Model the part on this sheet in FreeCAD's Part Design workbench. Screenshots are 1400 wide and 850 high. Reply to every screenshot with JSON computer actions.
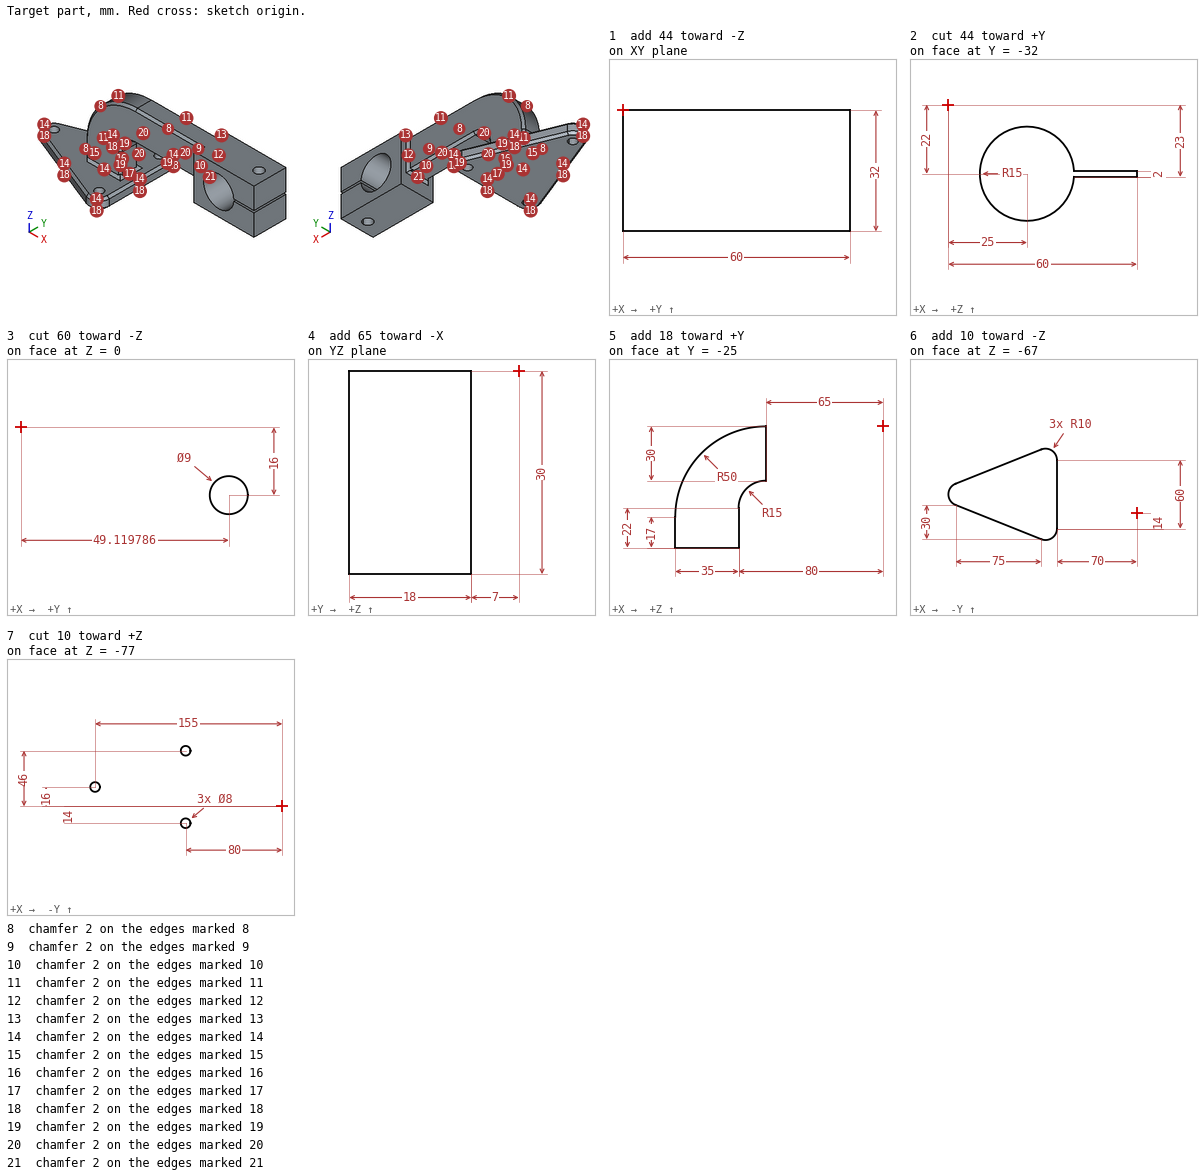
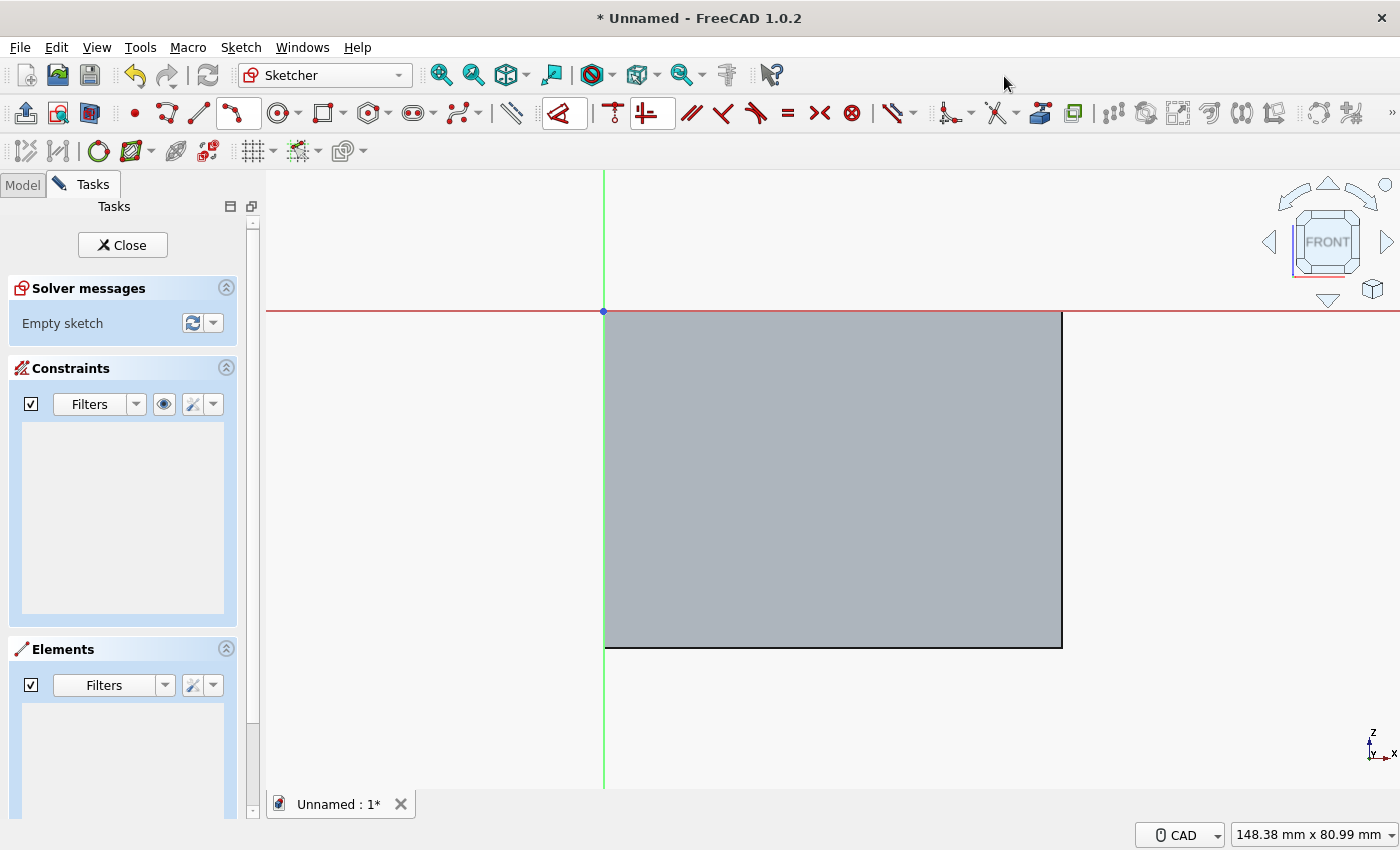
{"action": "scroll", "coordinate": [972, 236], "scroll_direction": "up", "scroll_amount": 2}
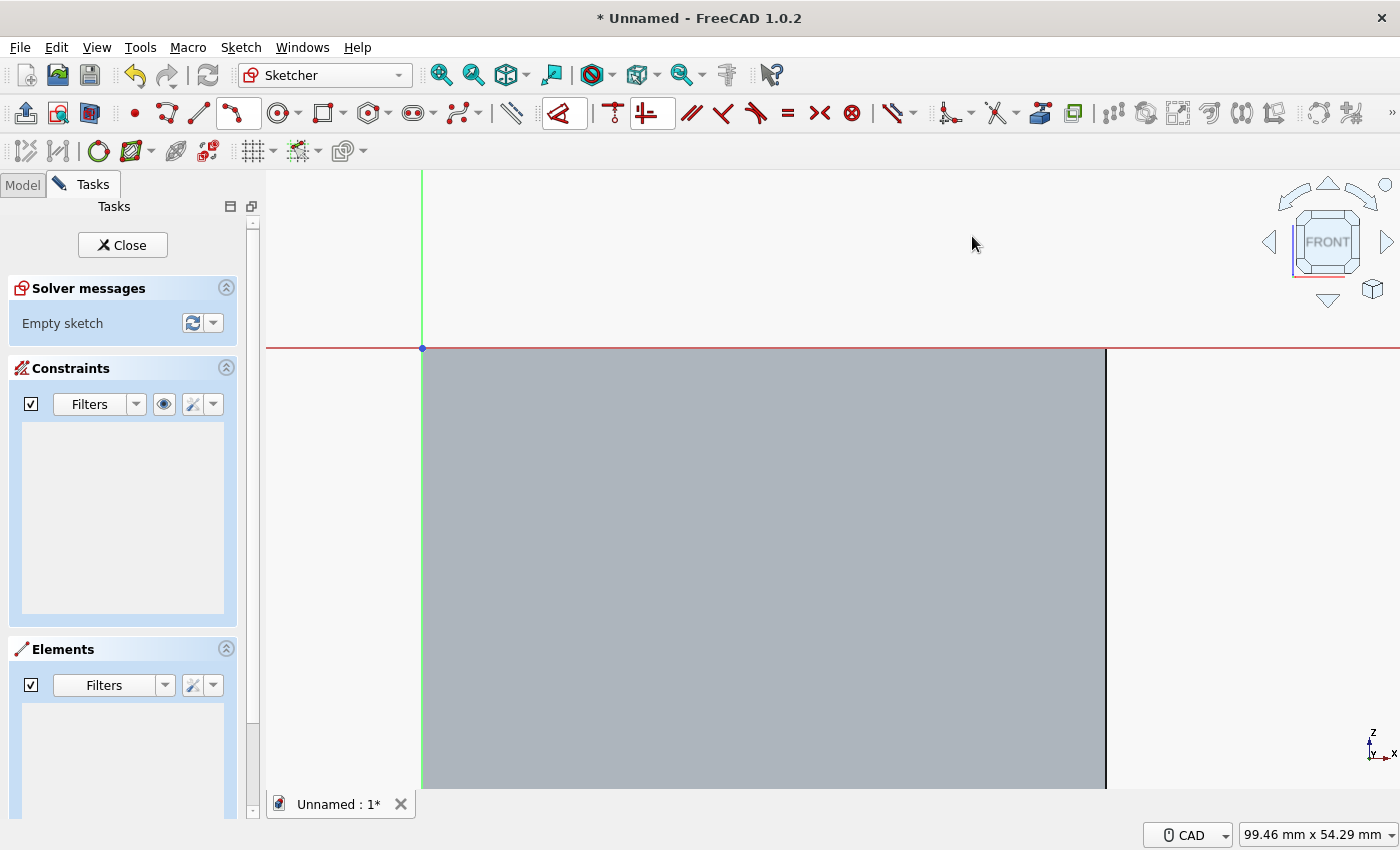
{"action": "left_click", "coordinate": [168, 114]}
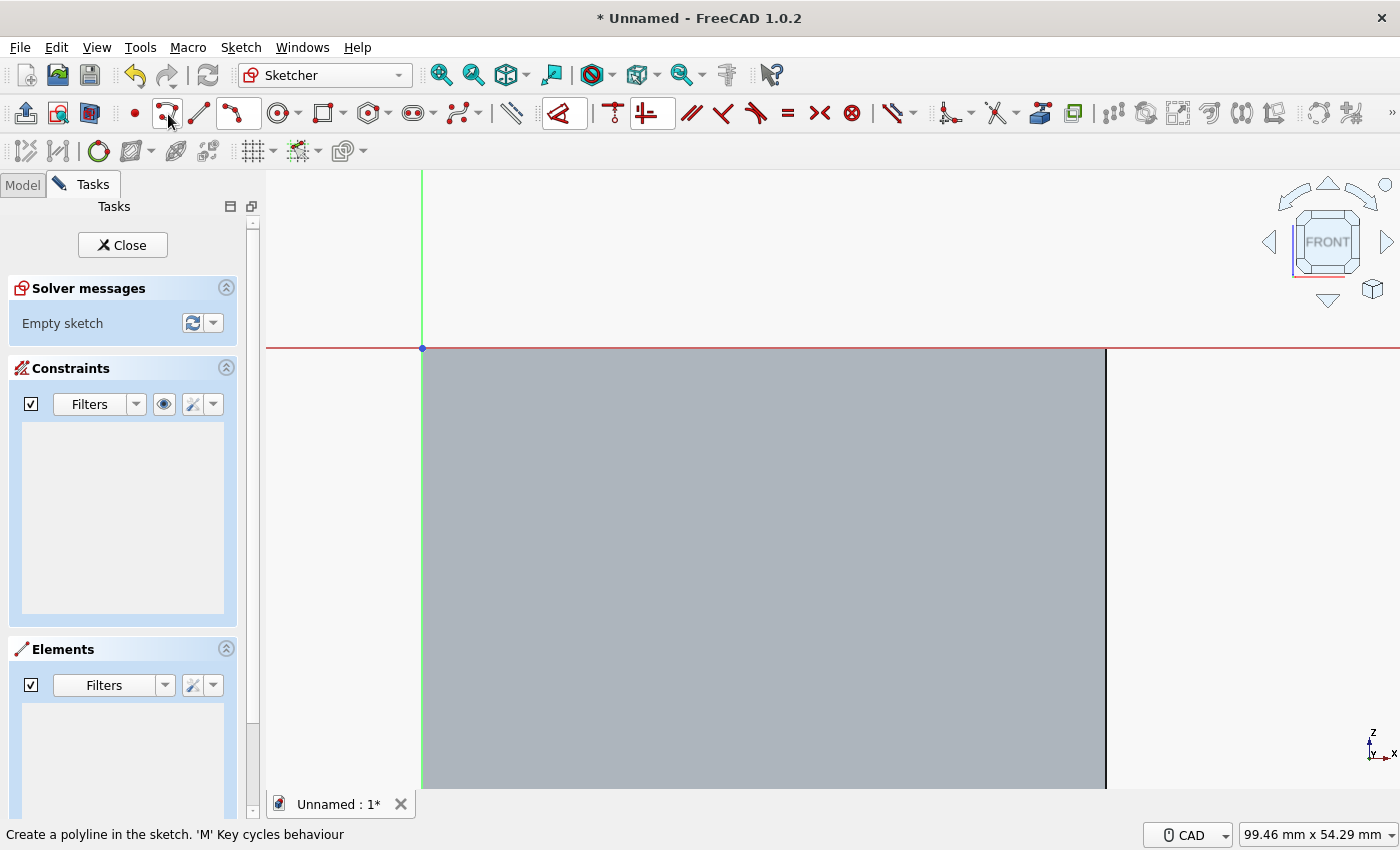
{"action": "left_click", "coordinate": [878, 611]}
{"action": "left_click", "coordinate": [1106, 611]}
{"action": "left_click", "coordinate": [1106, 588]}
{"action": "left_click", "coordinate": [878, 588]}
{"action": "right_click", "coordinate": [878, 588]}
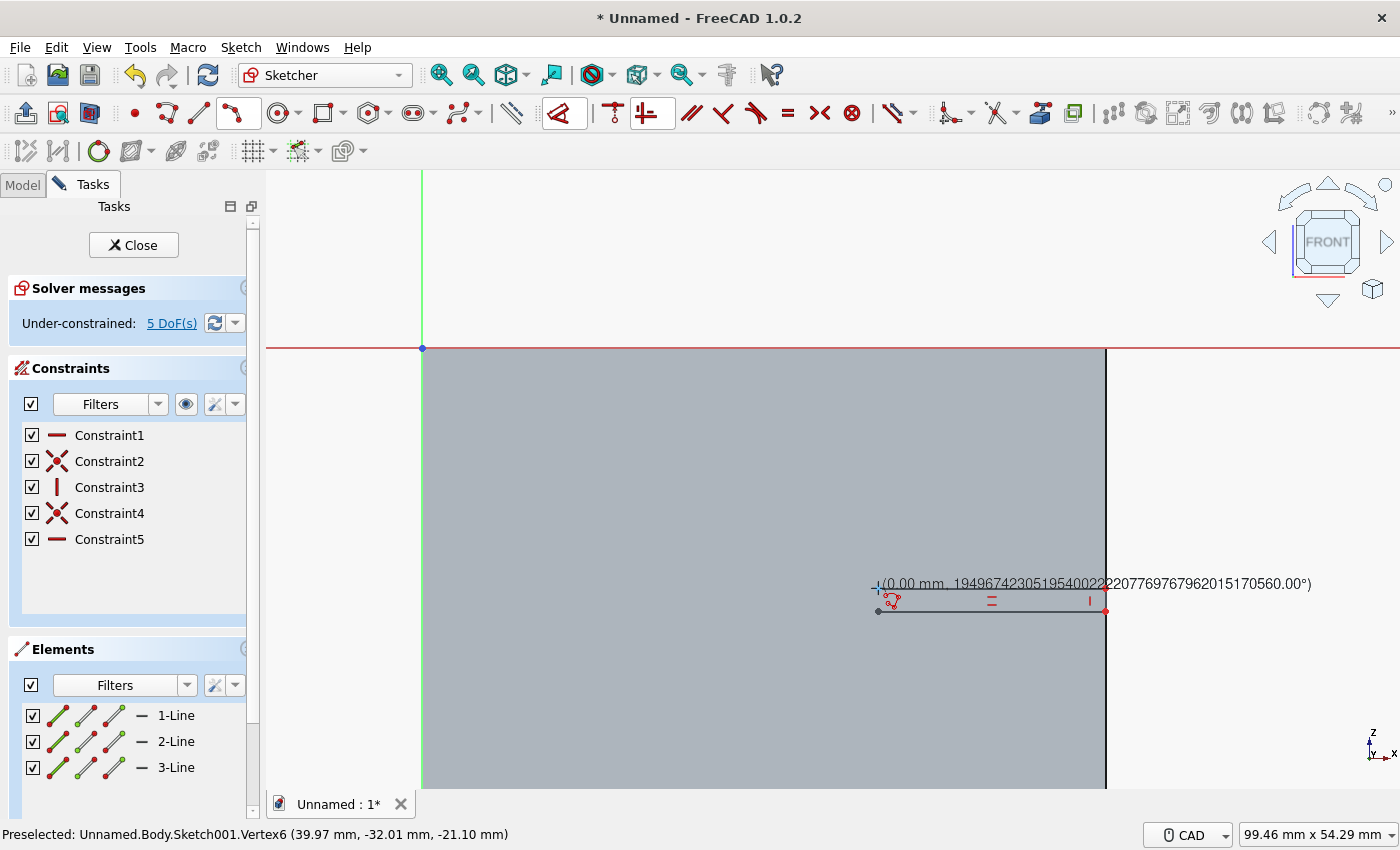
{"action": "left_click", "coordinate": [232, 114]}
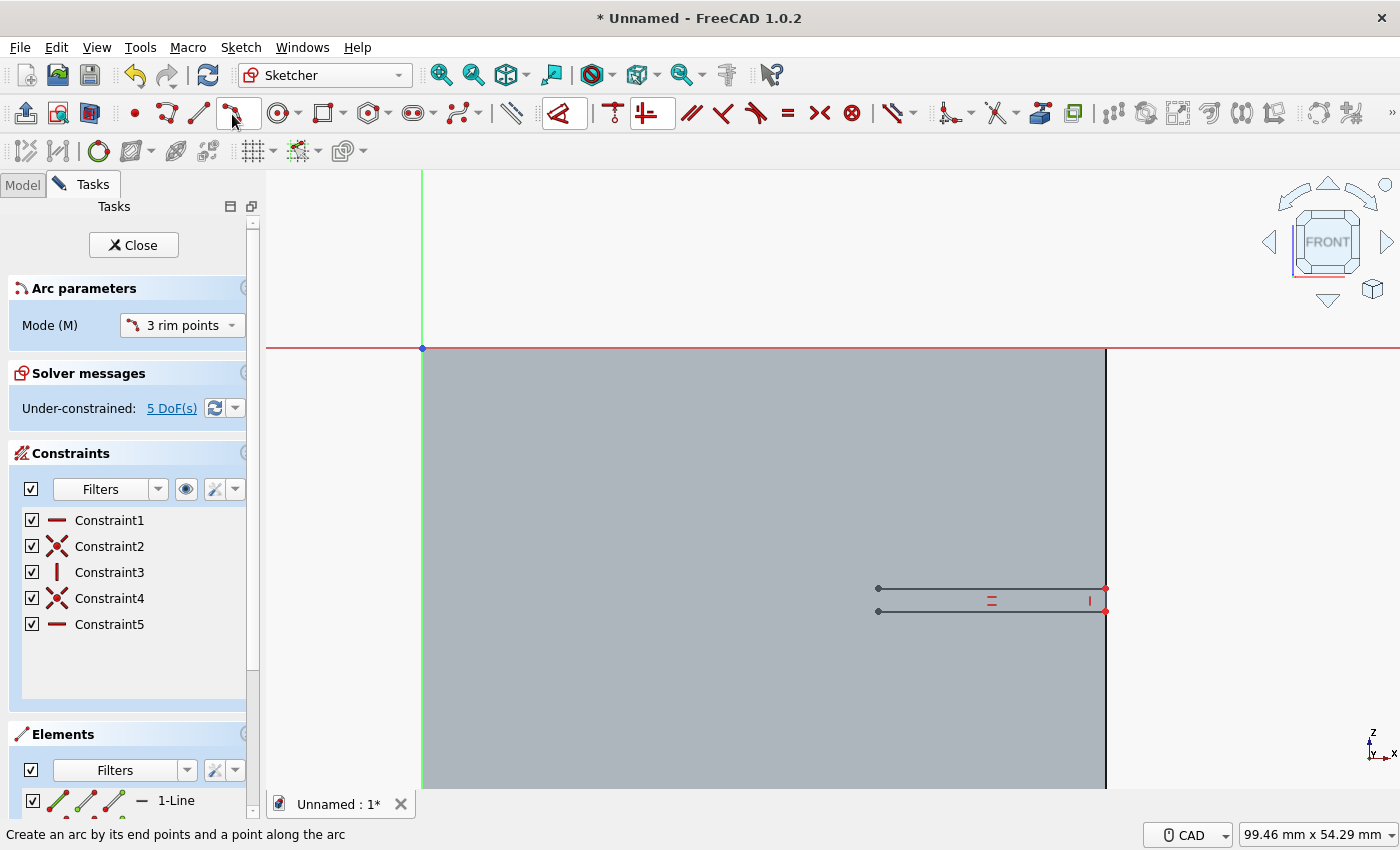
{"action": "left_click", "coordinate": [878, 589]}
{"action": "left_click", "coordinate": [878, 612]}
{"action": "left_click", "coordinate": [536, 599]}
{"action": "key", "text": "Escape"}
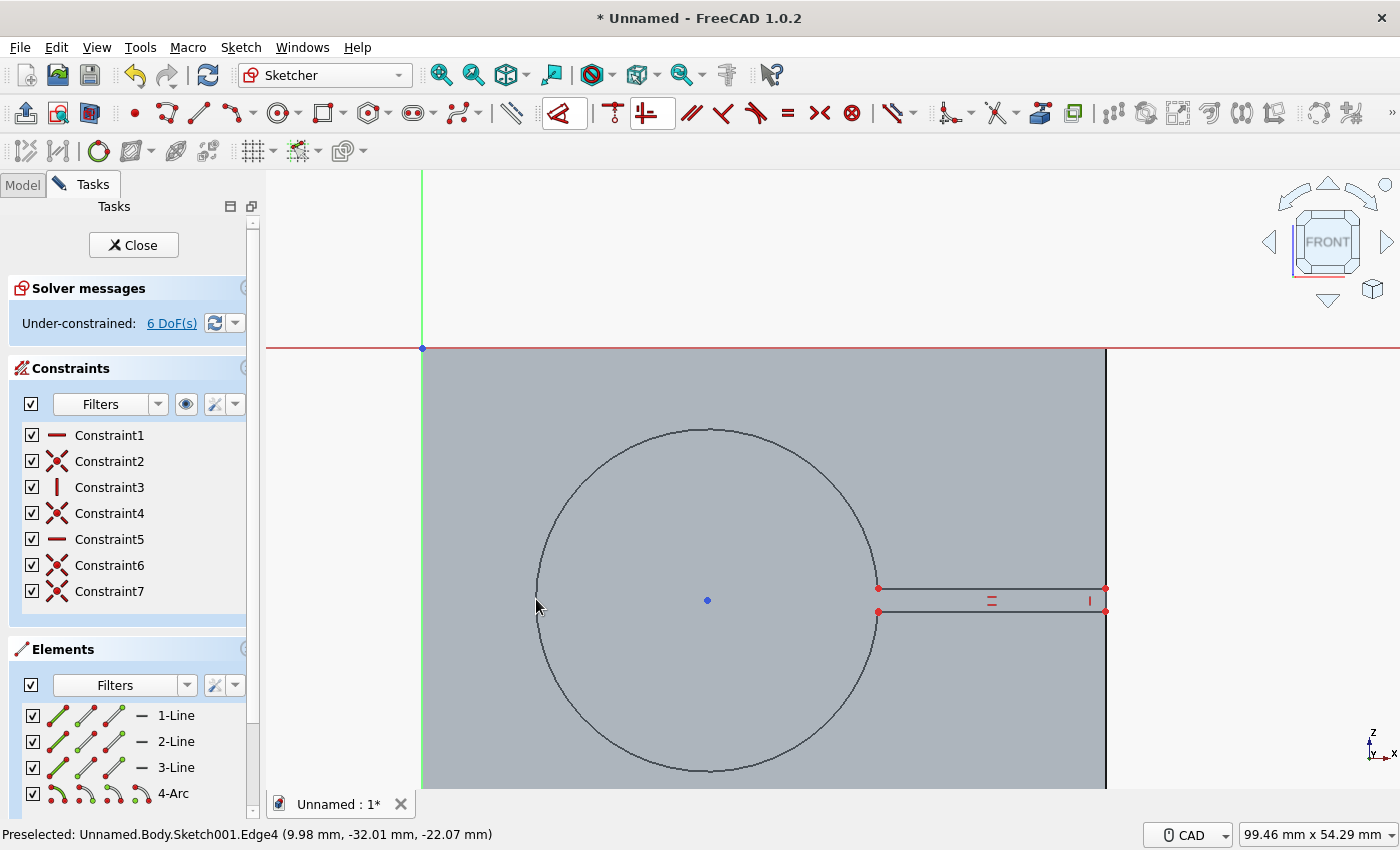
{"action": "left_click", "coordinate": [558, 114]}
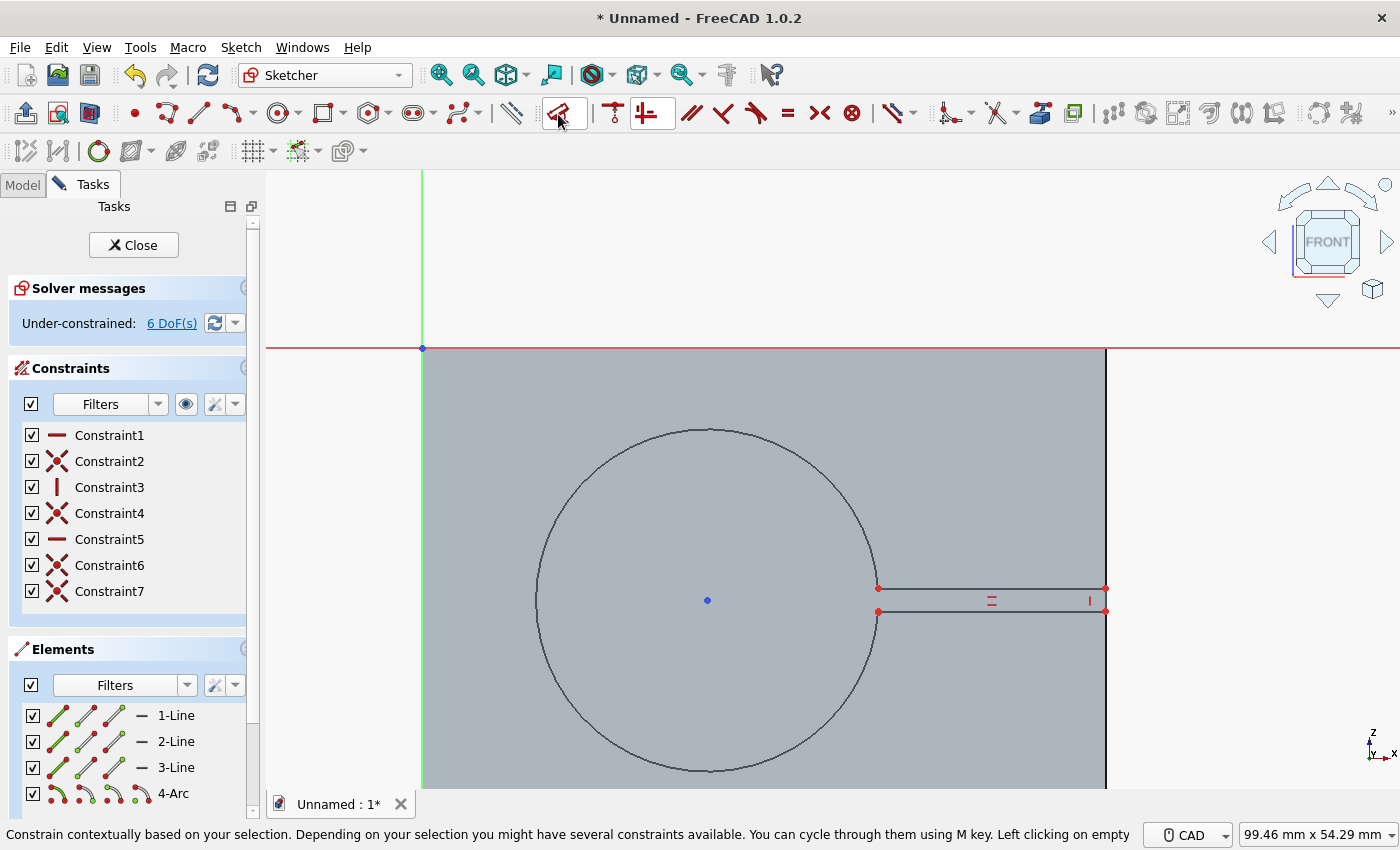
{"action": "left_click", "coordinate": [650, 439]}
{"action": "left_click", "coordinate": [639, 409]}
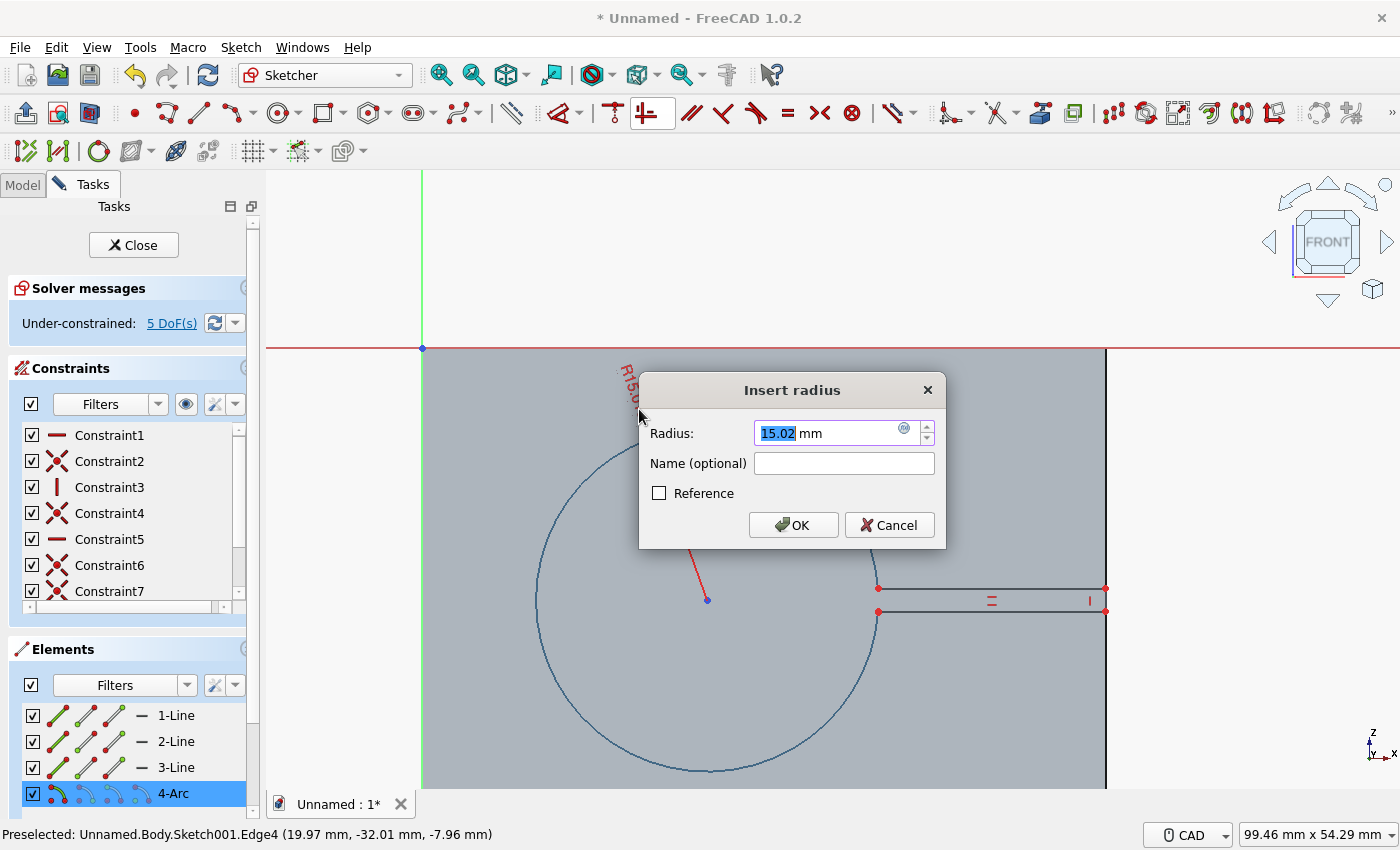
{"action": "type", "text": "15"}
{"action": "key", "text": "Return"}